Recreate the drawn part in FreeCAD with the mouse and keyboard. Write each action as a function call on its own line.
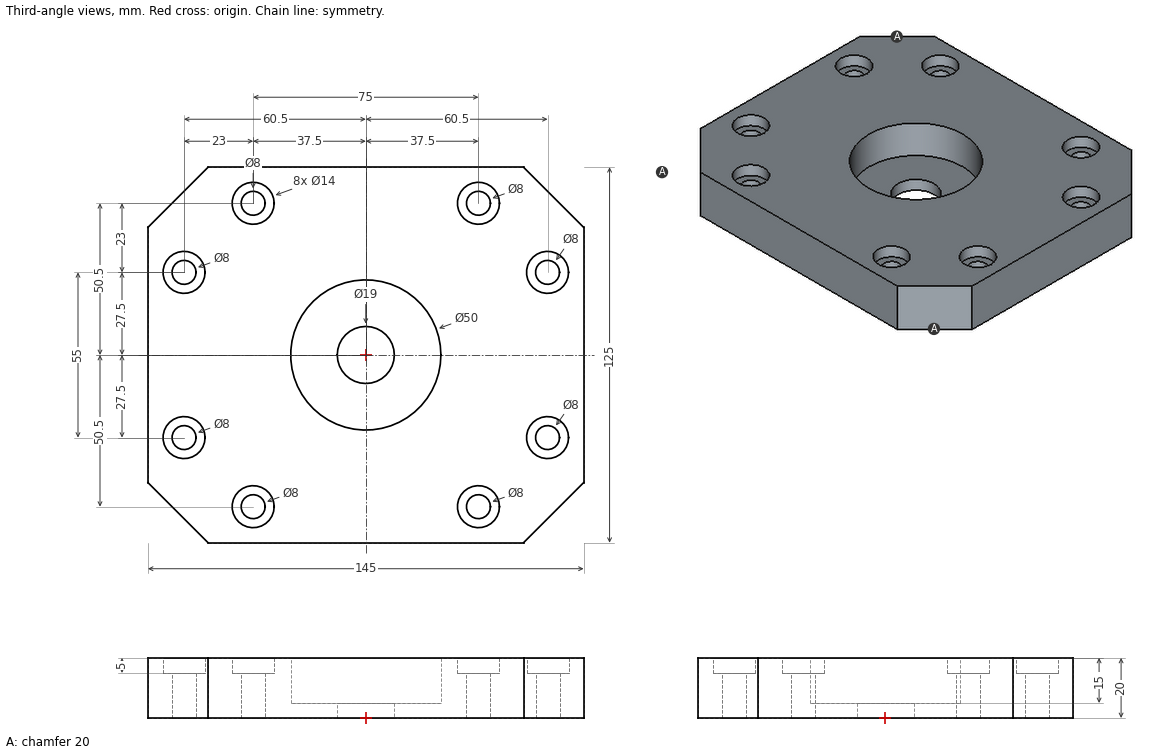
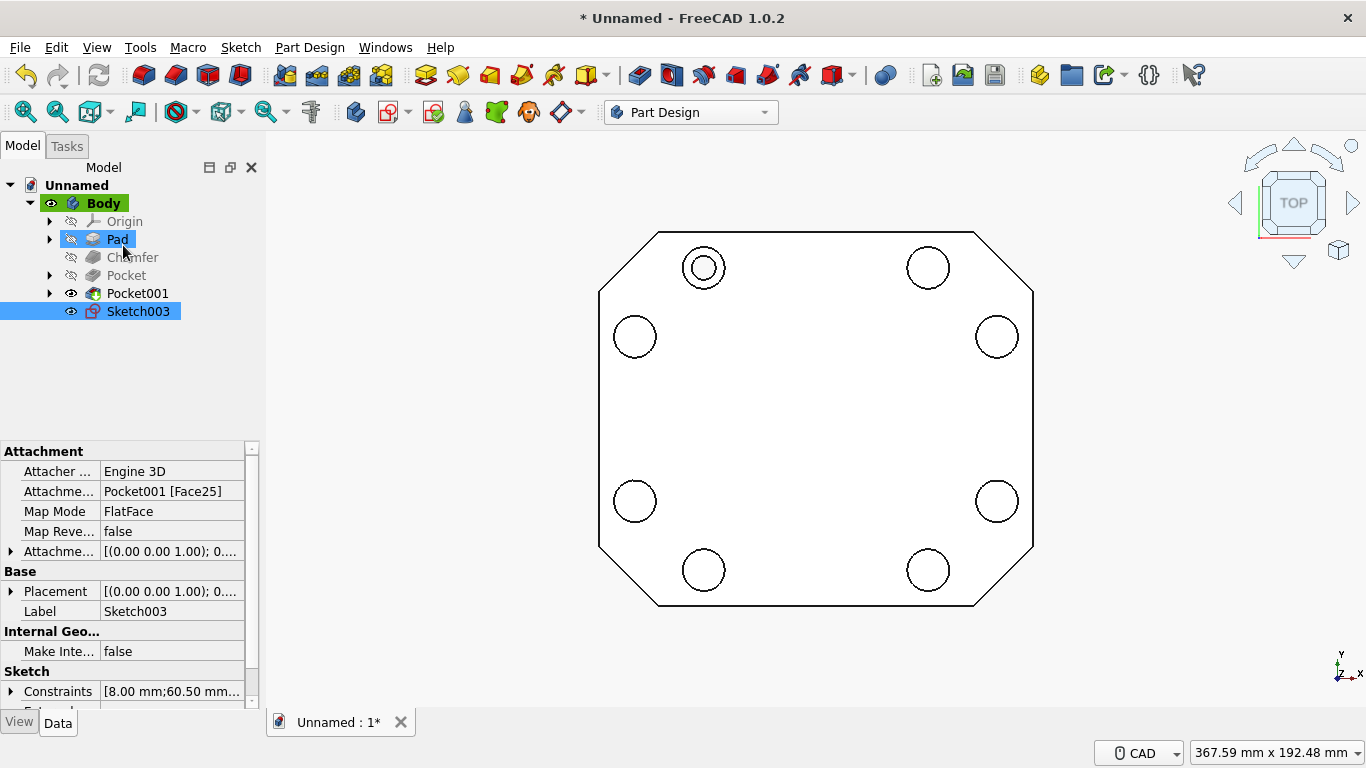
click(640, 76)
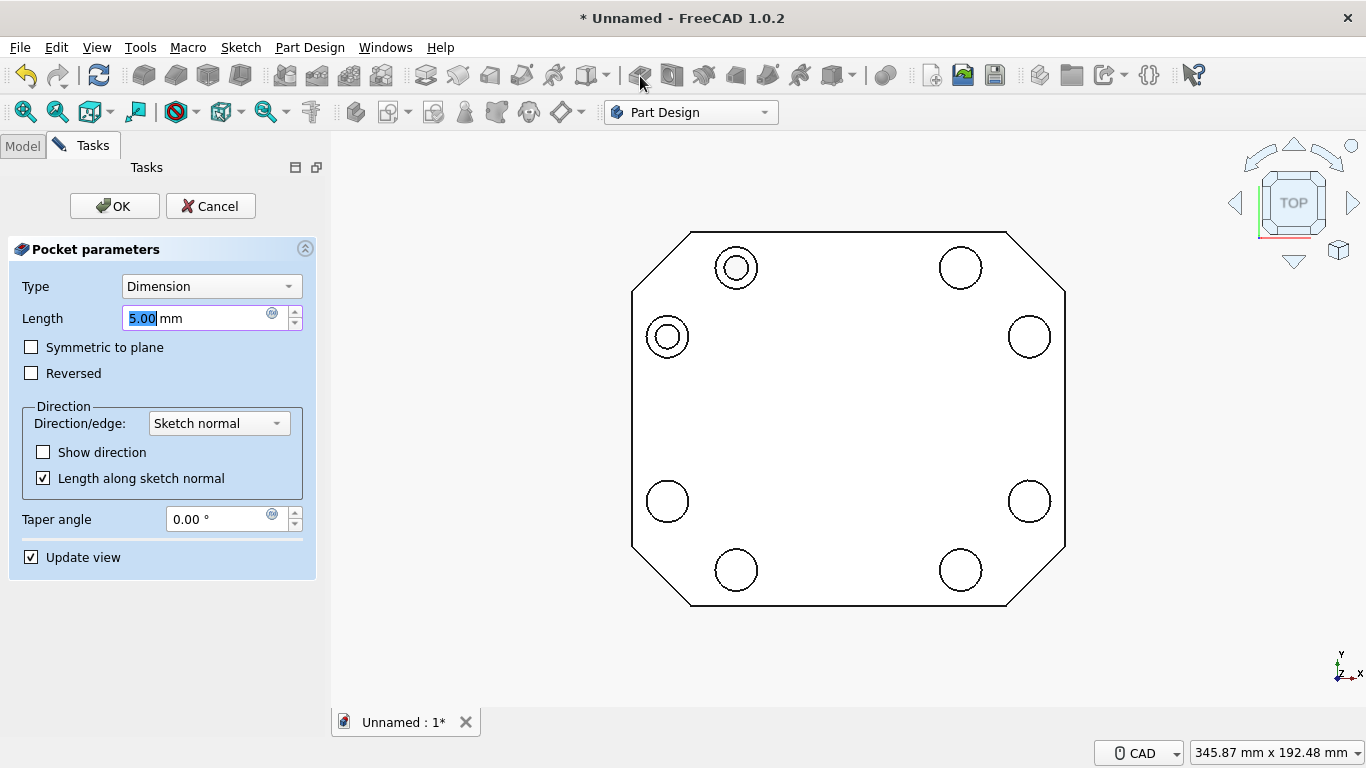
click(212, 286)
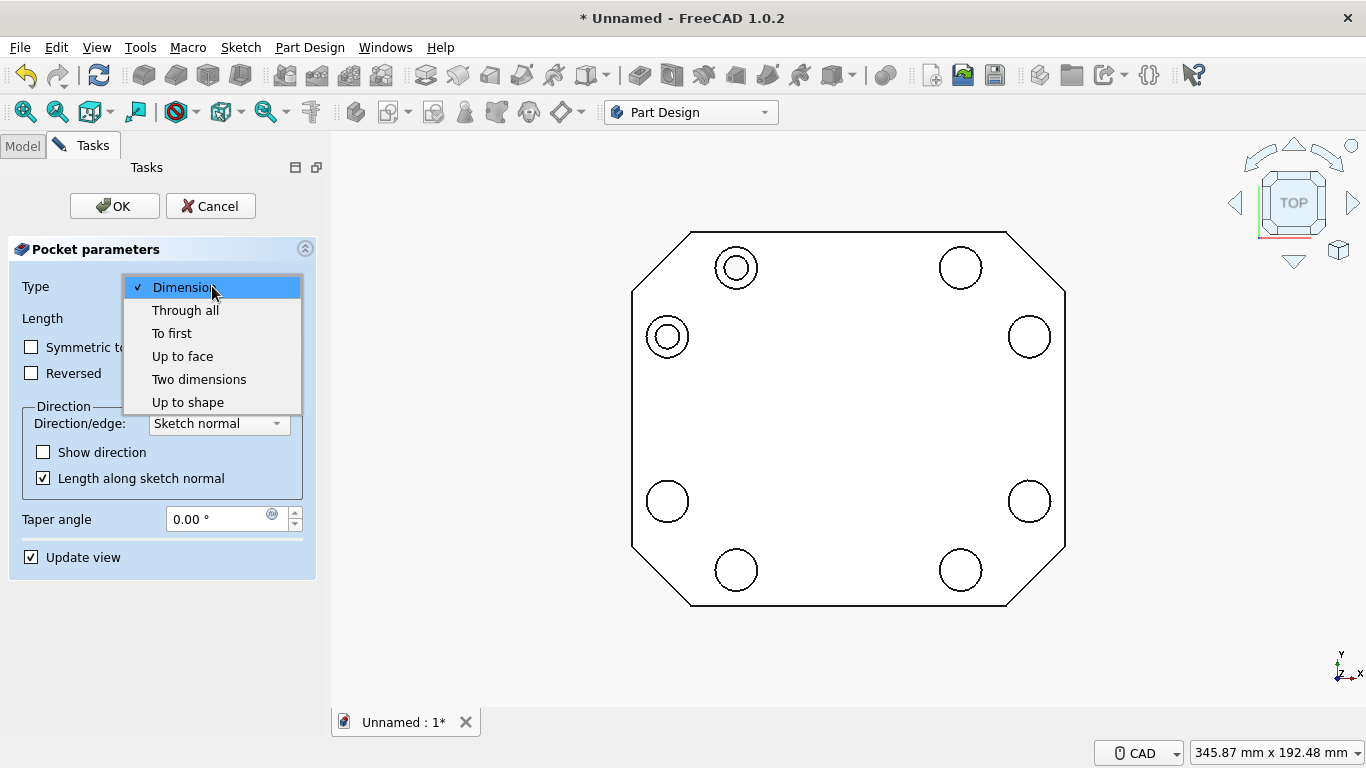
click(212, 334)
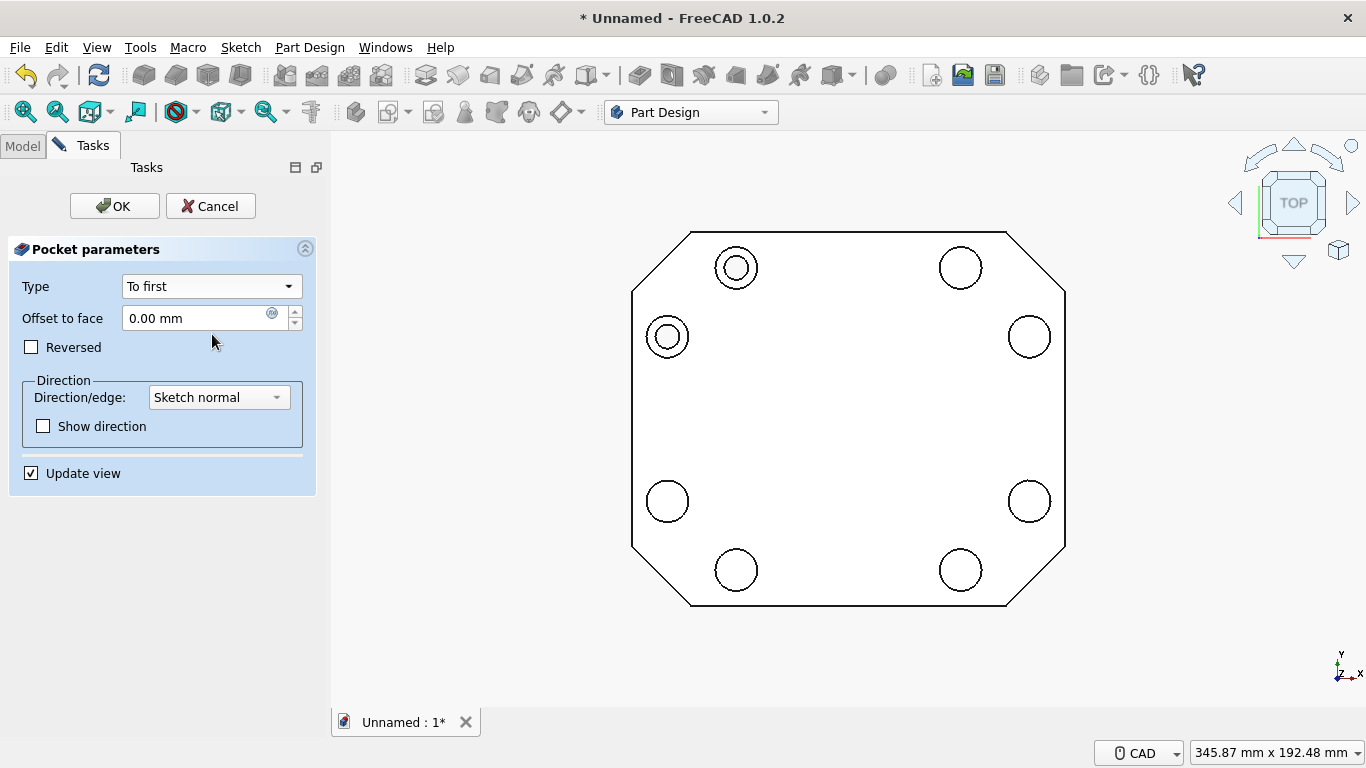
click(115, 206)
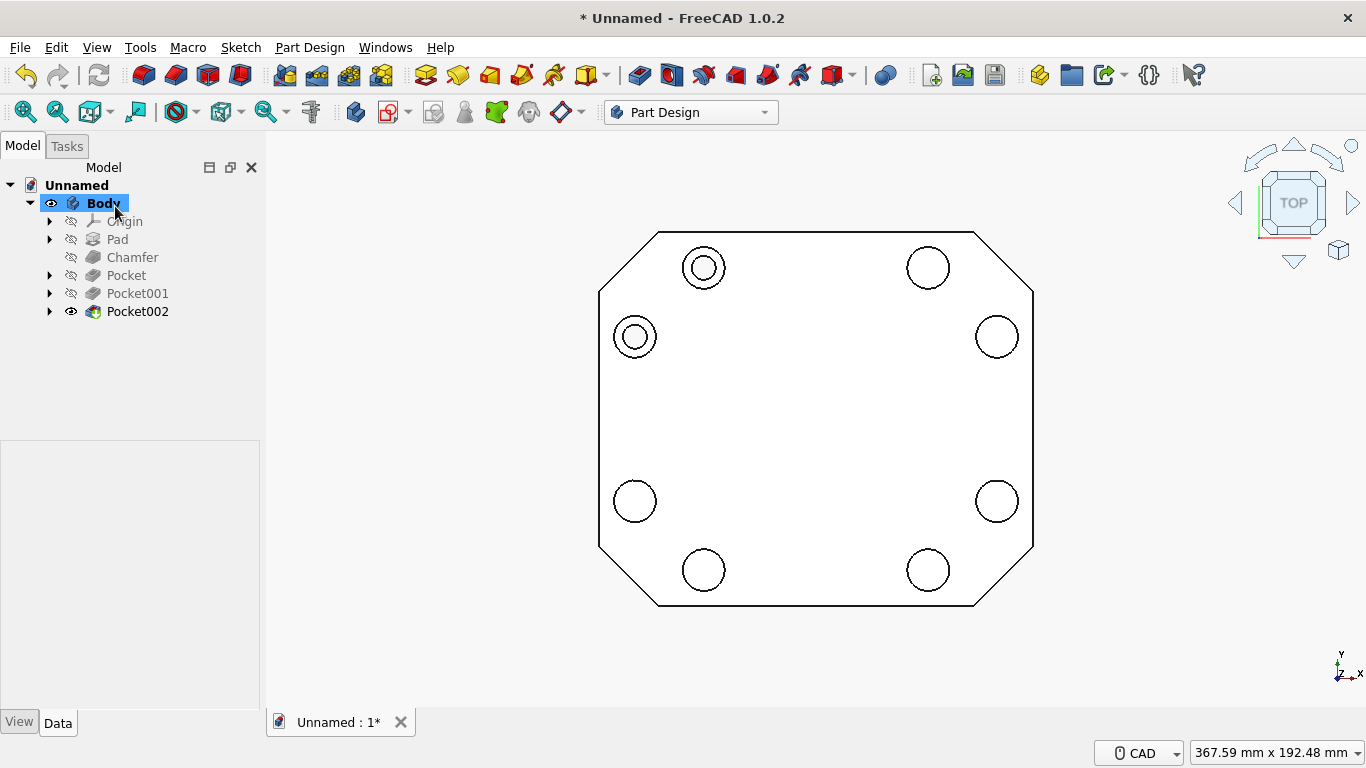
click(635, 500)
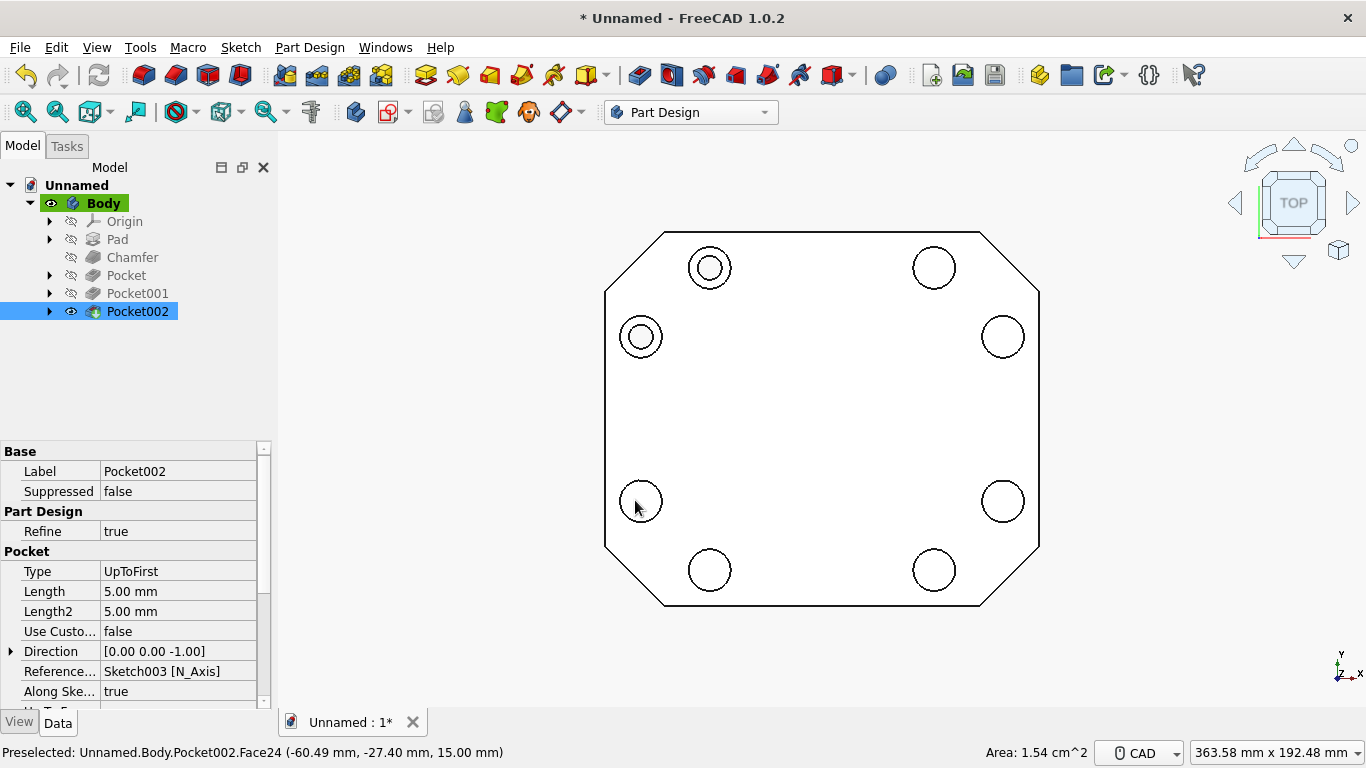
click(388, 112)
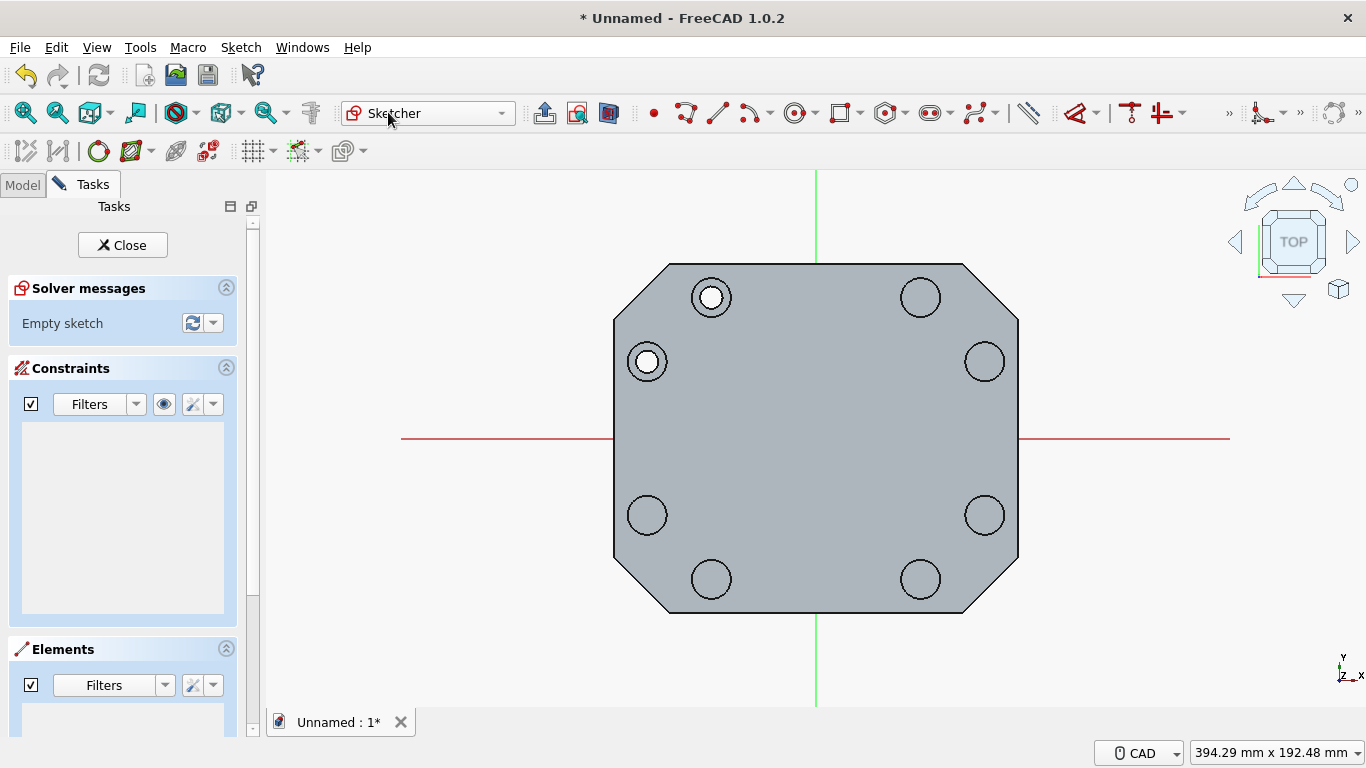
click(610, 114)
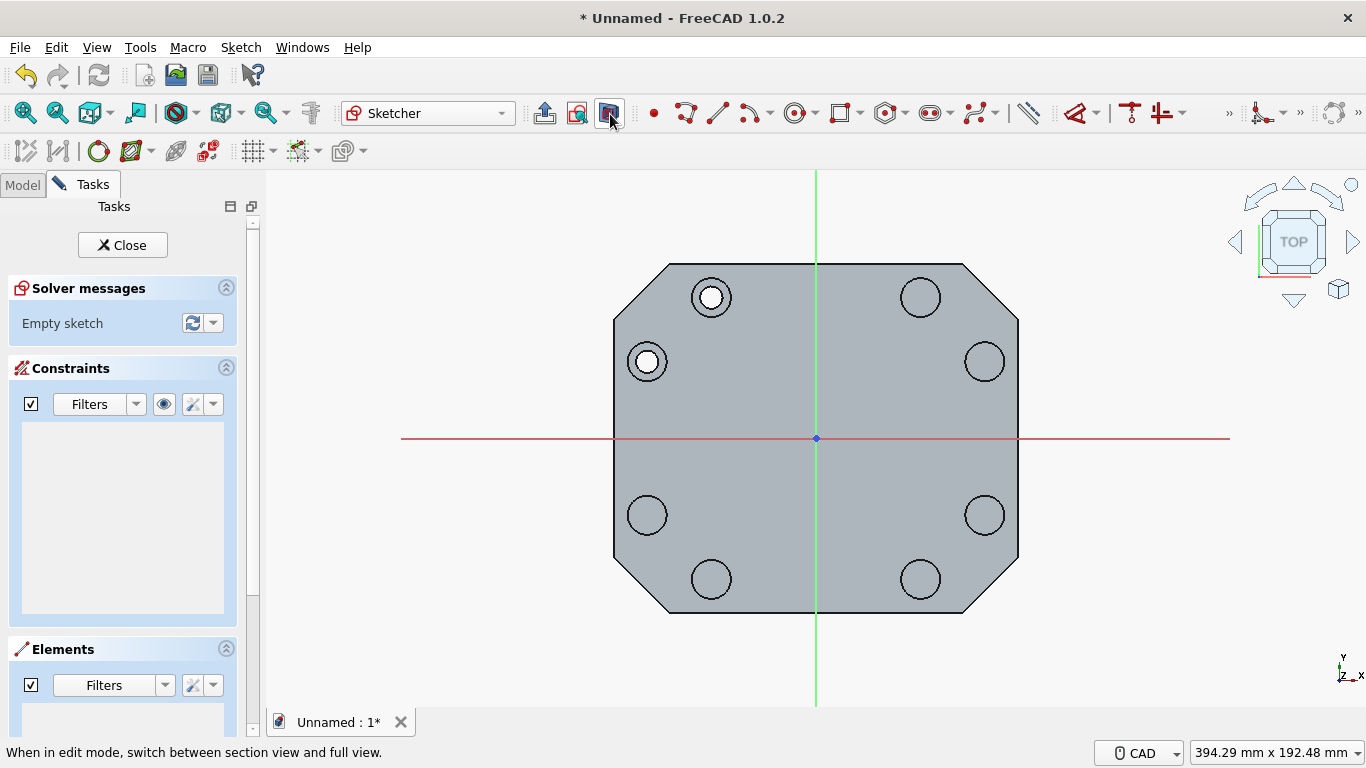
scroll(641, 520, up, 14)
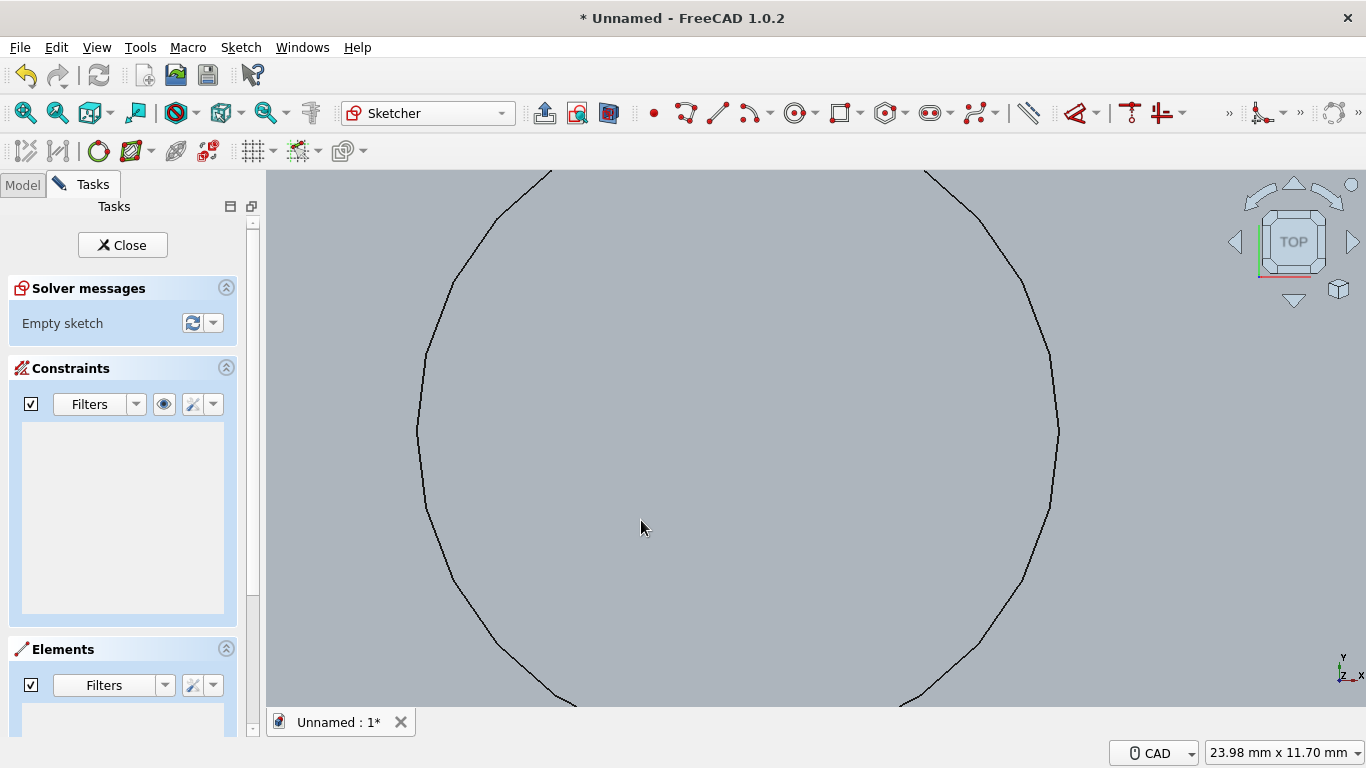
click(796, 114)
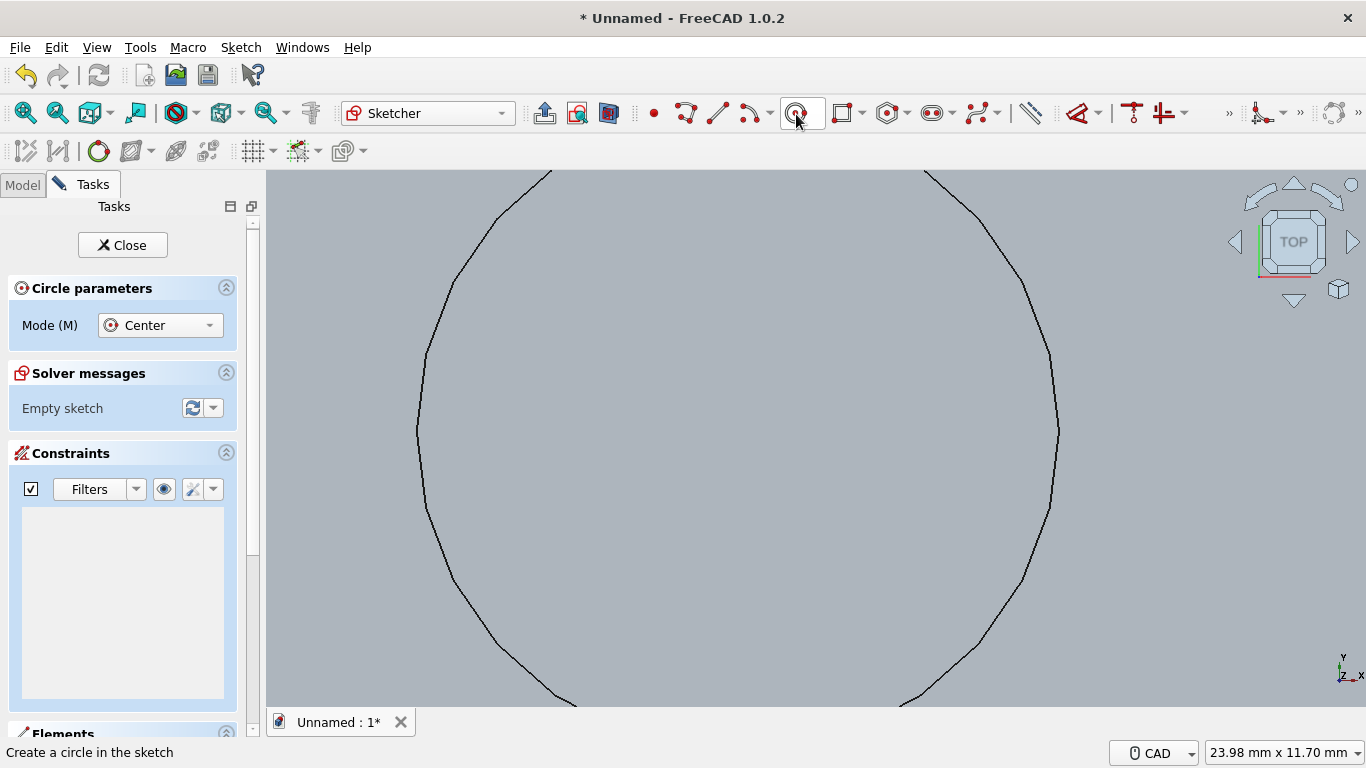
click(738, 431)
click(868, 302)
key(Escape)